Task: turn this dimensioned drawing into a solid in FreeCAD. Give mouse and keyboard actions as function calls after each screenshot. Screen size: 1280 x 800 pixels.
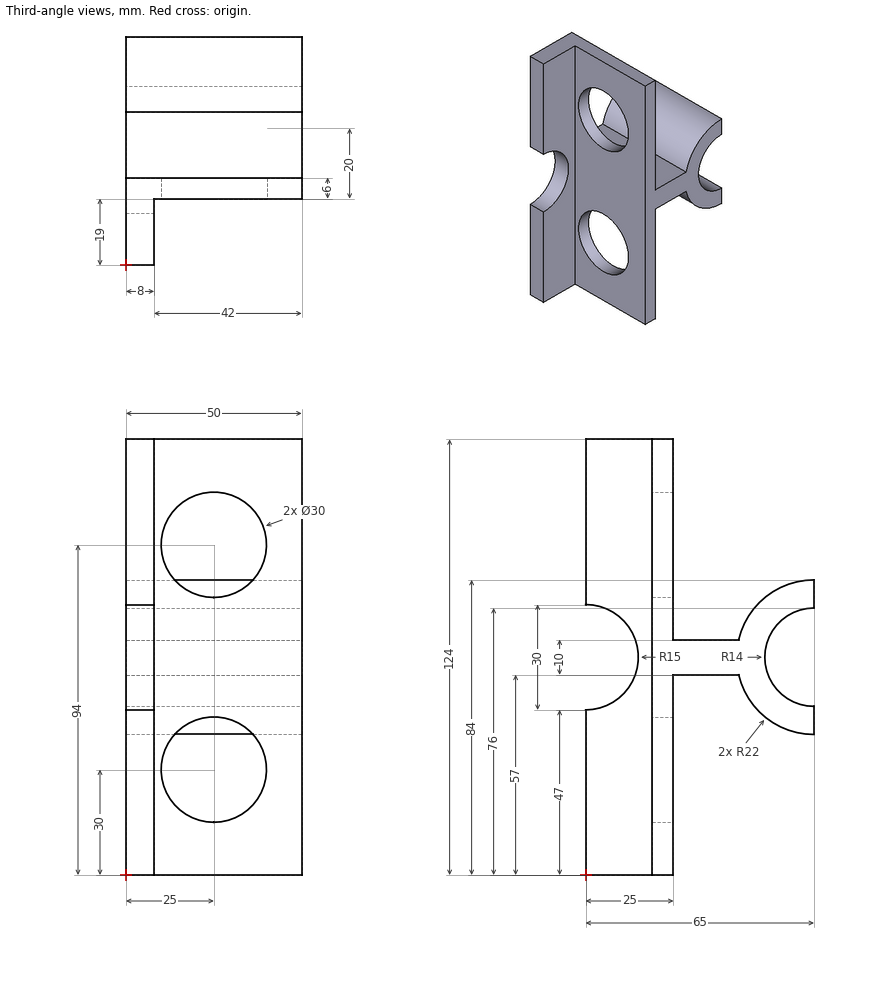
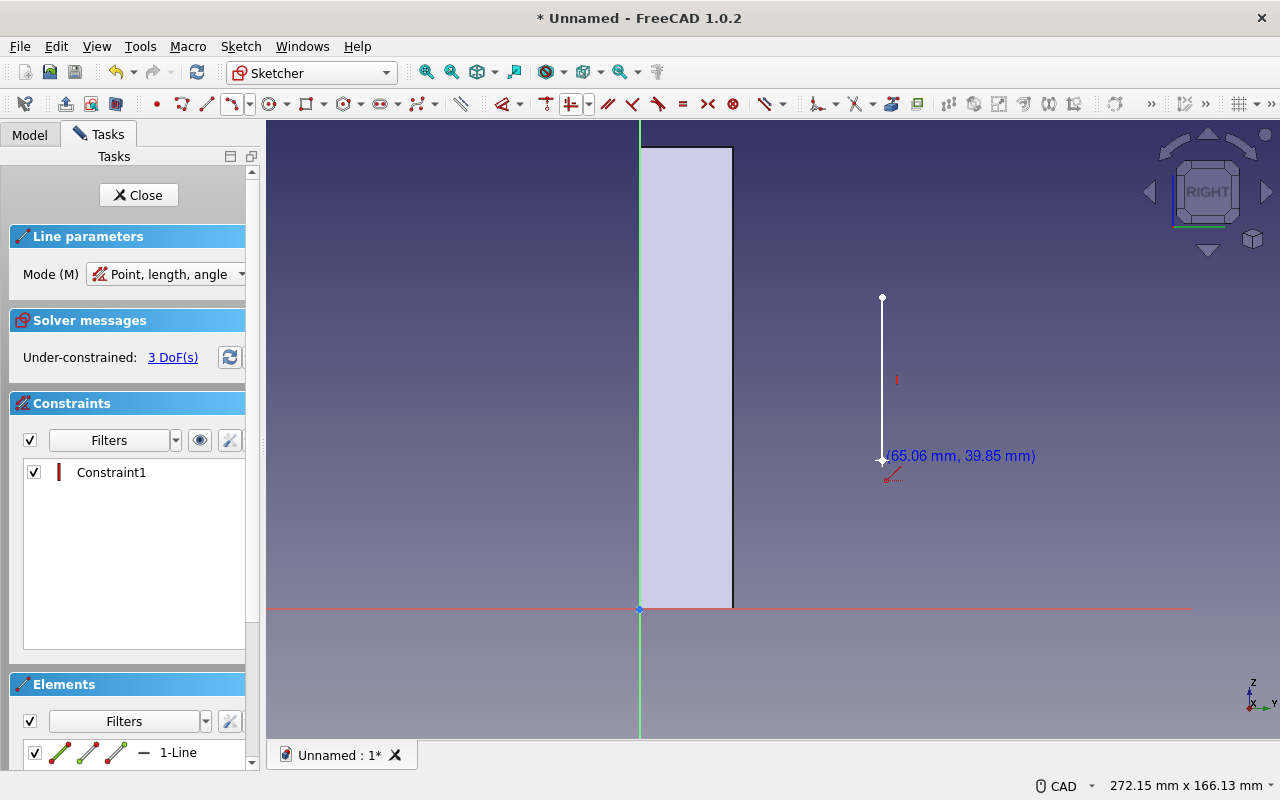
key(g)
key(m)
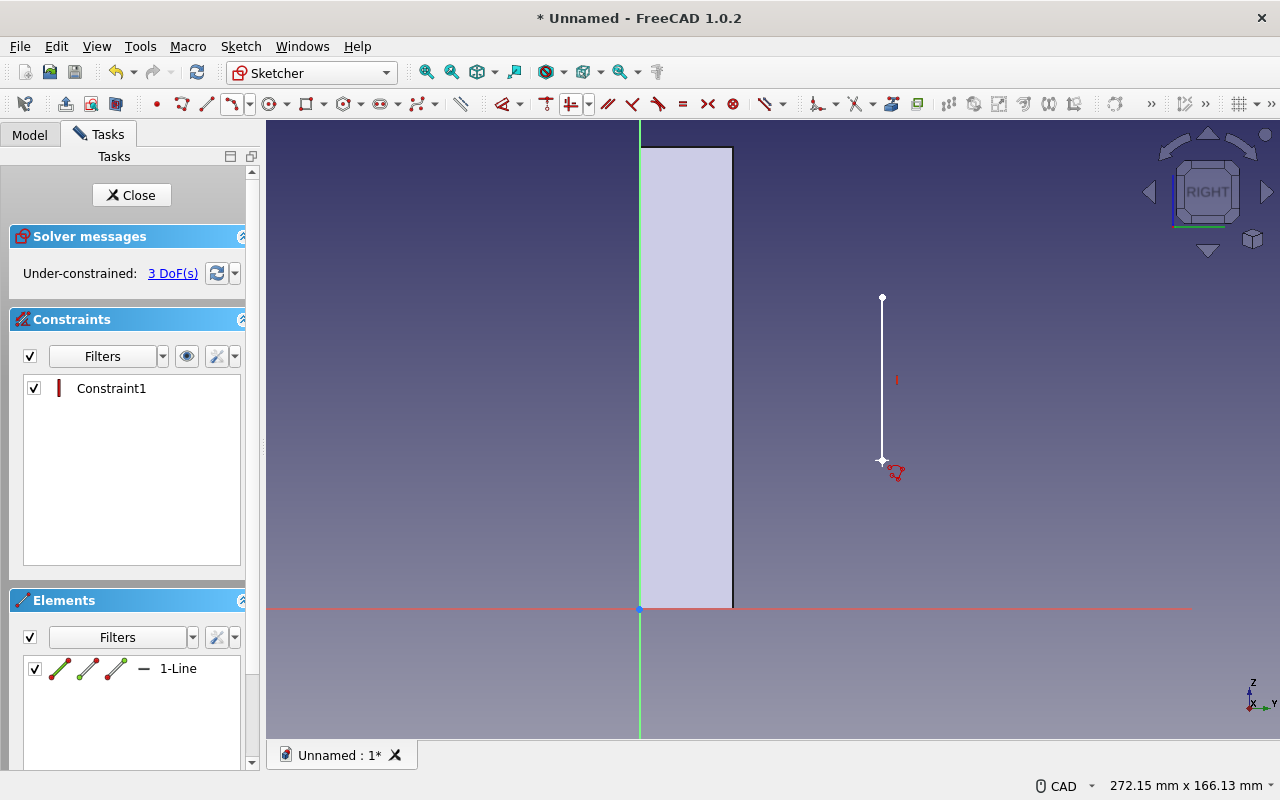
click(802, 397)
click(733, 397)
click(733, 360)
click(802, 360)
right_click(802, 360)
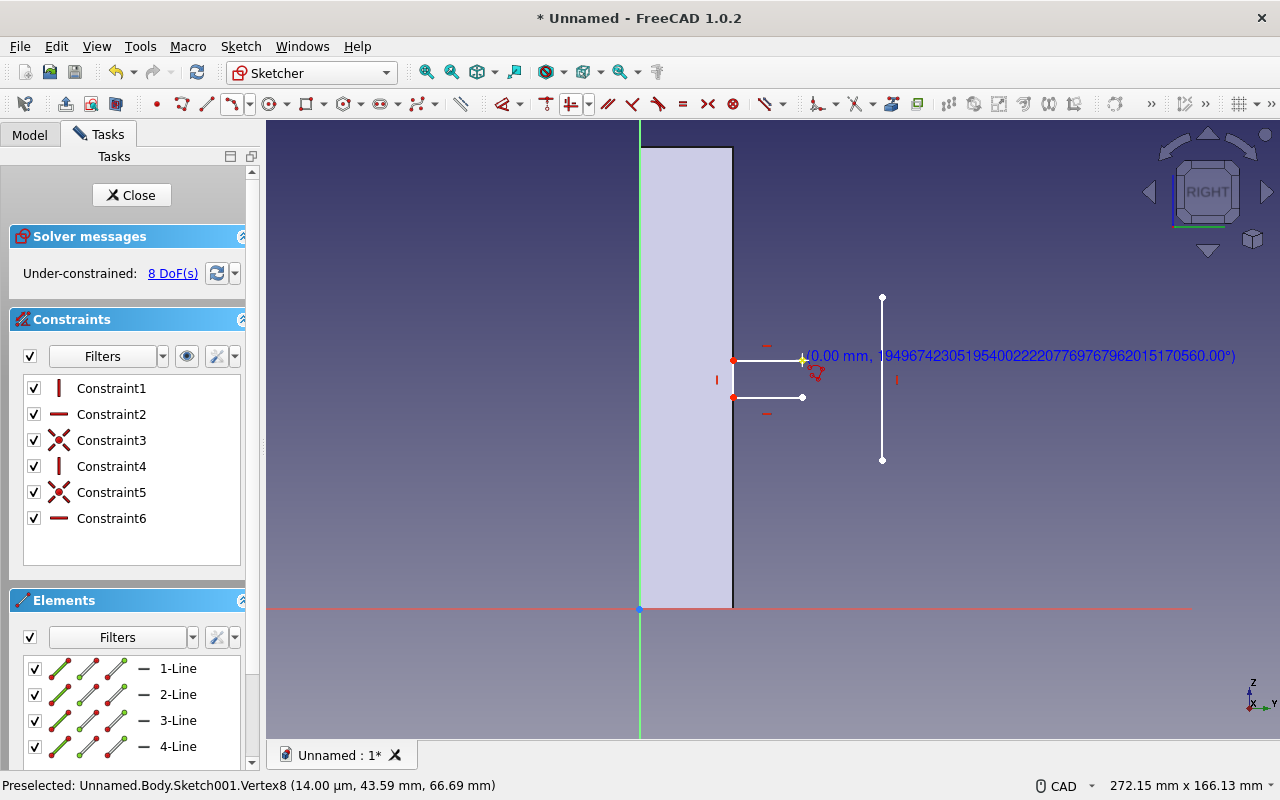
key(g)
key(3)
key(a)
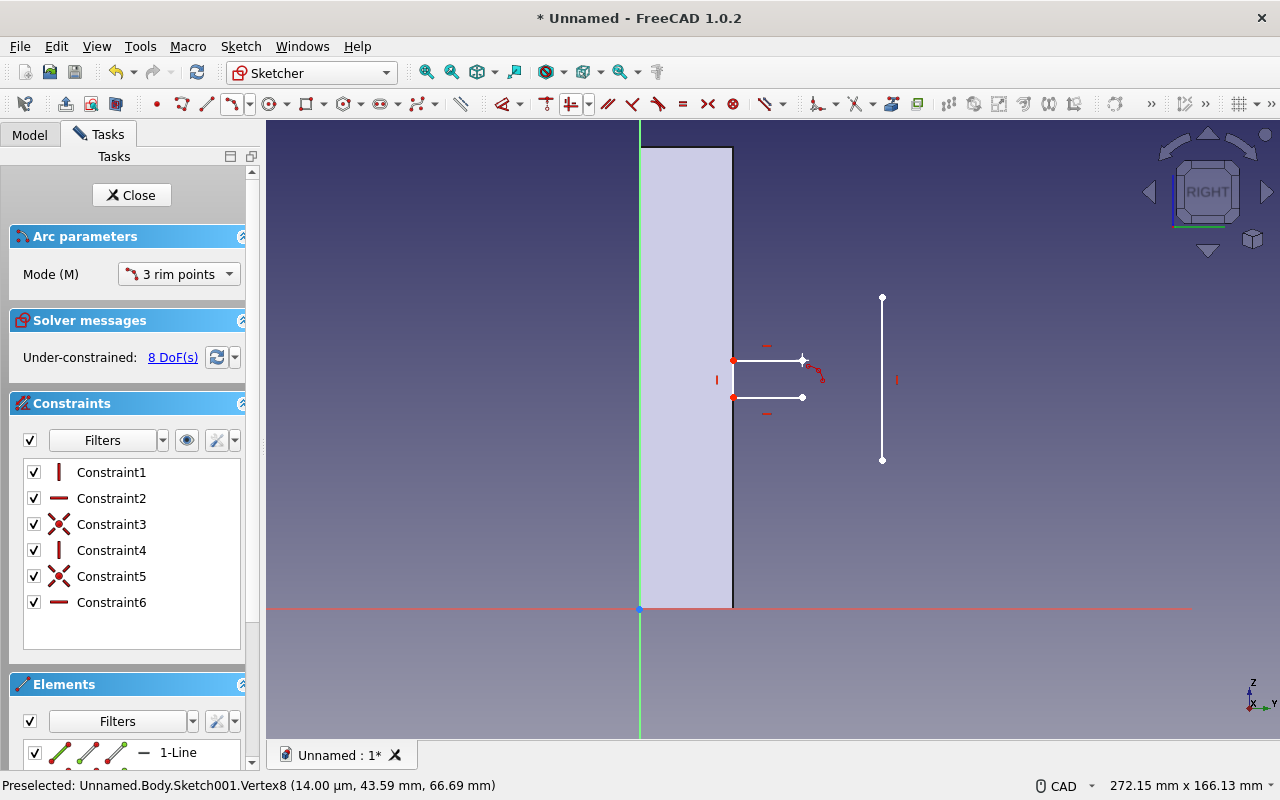
click(882, 461)
click(802, 398)
click(831, 443)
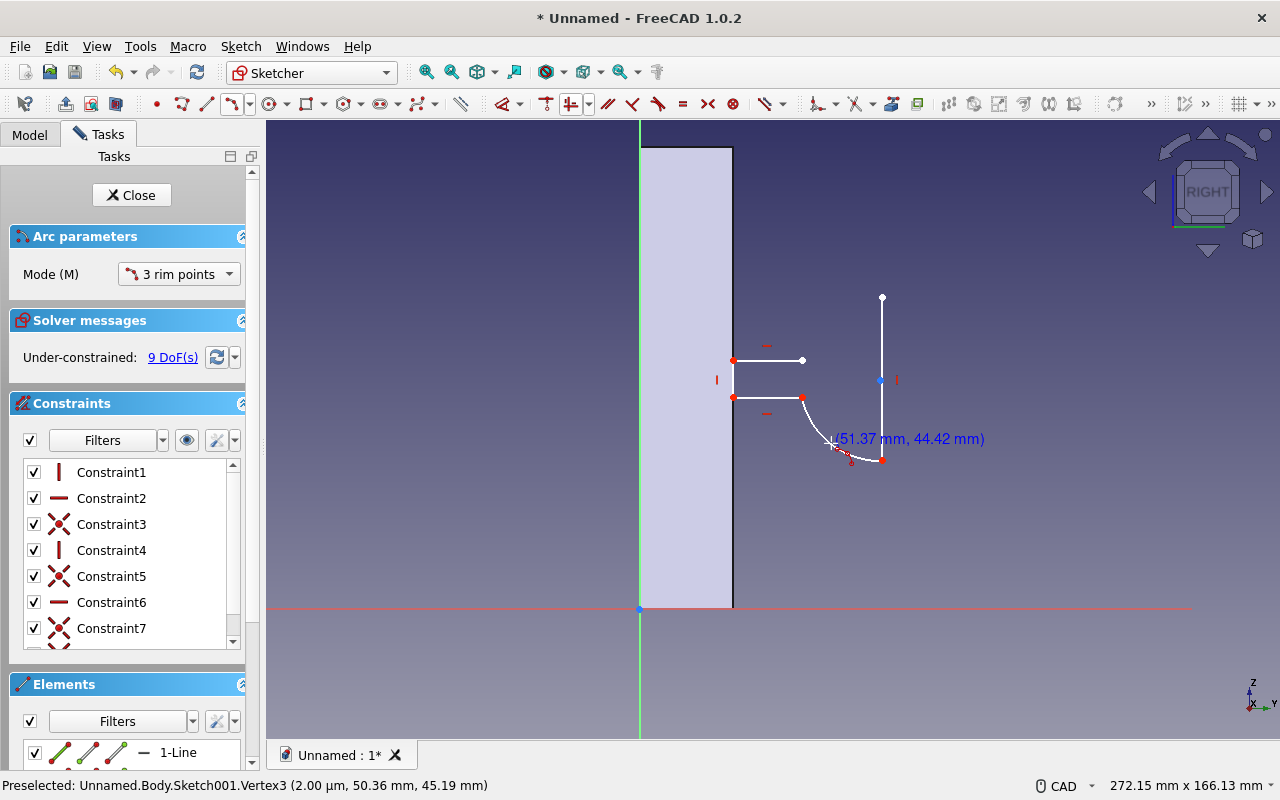
click(802, 361)
click(882, 298)
click(831, 314)
key(Escape)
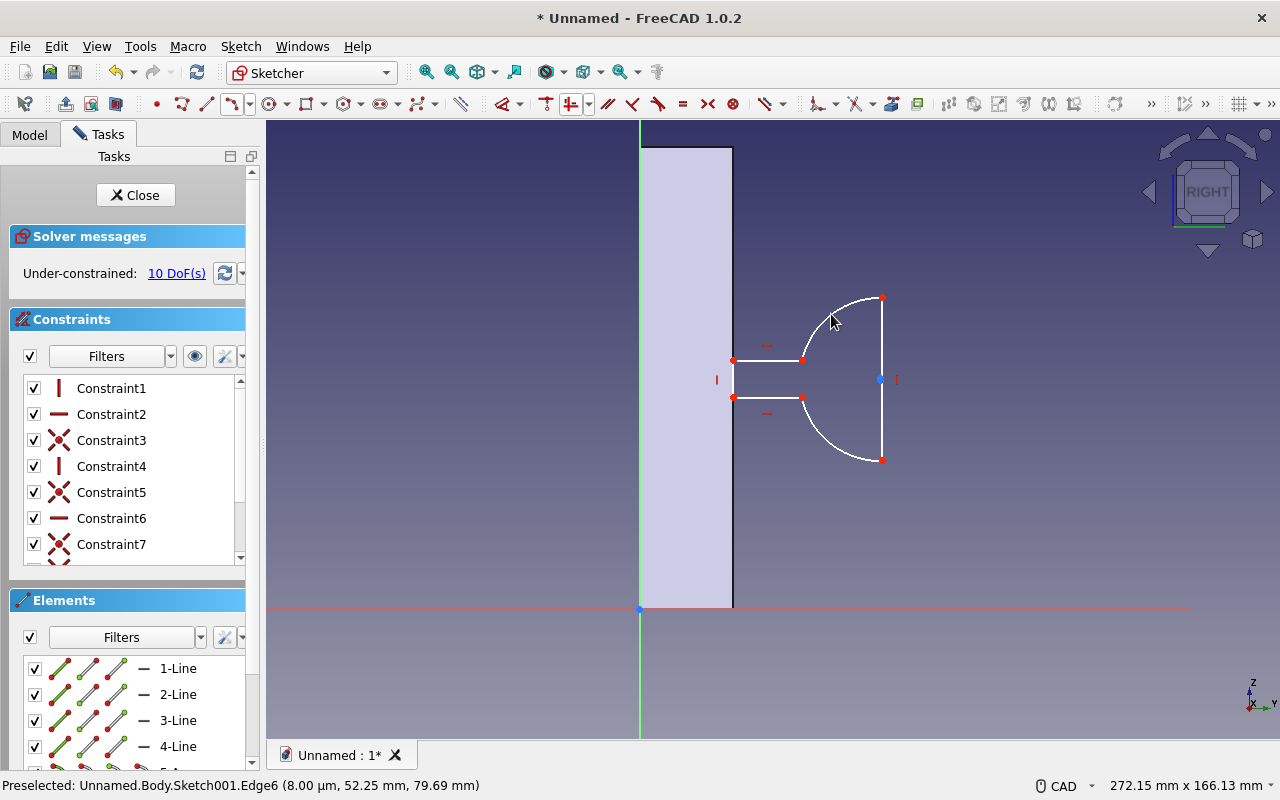
click(815, 428)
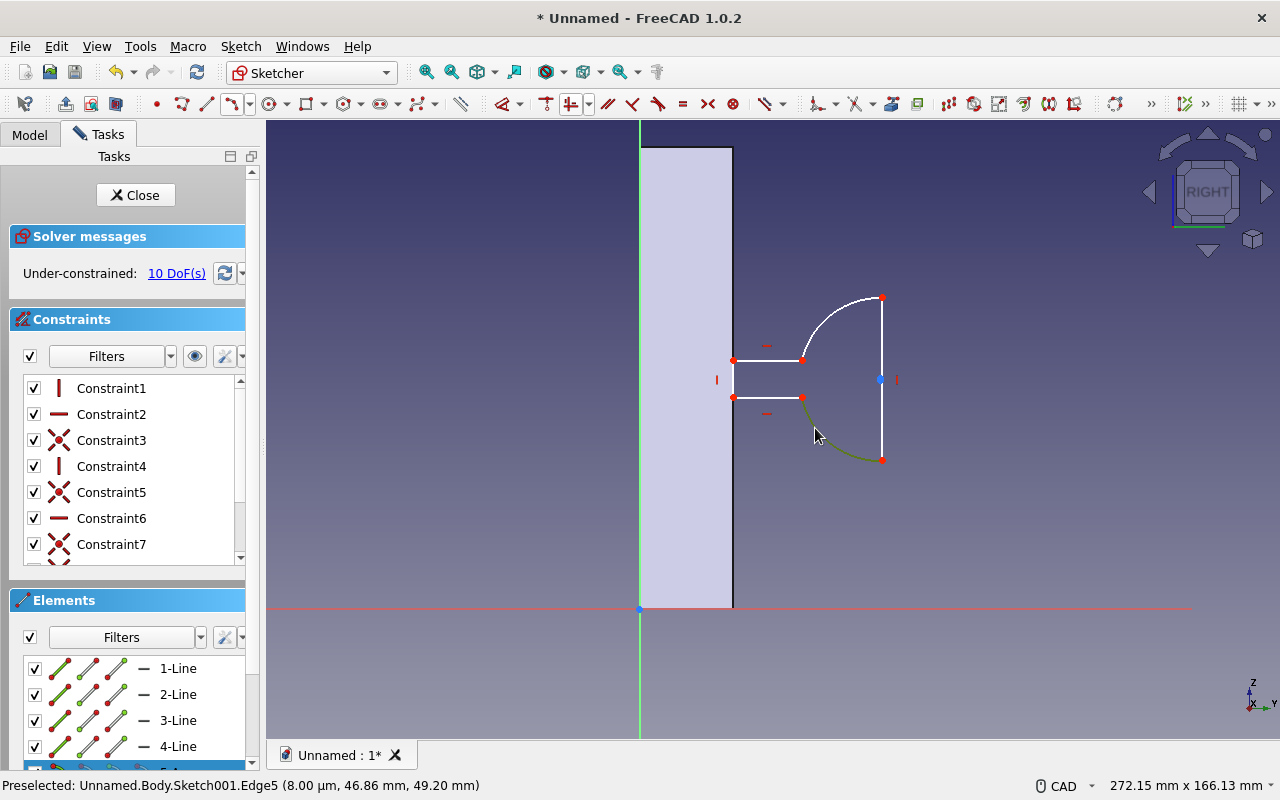
click(850, 304)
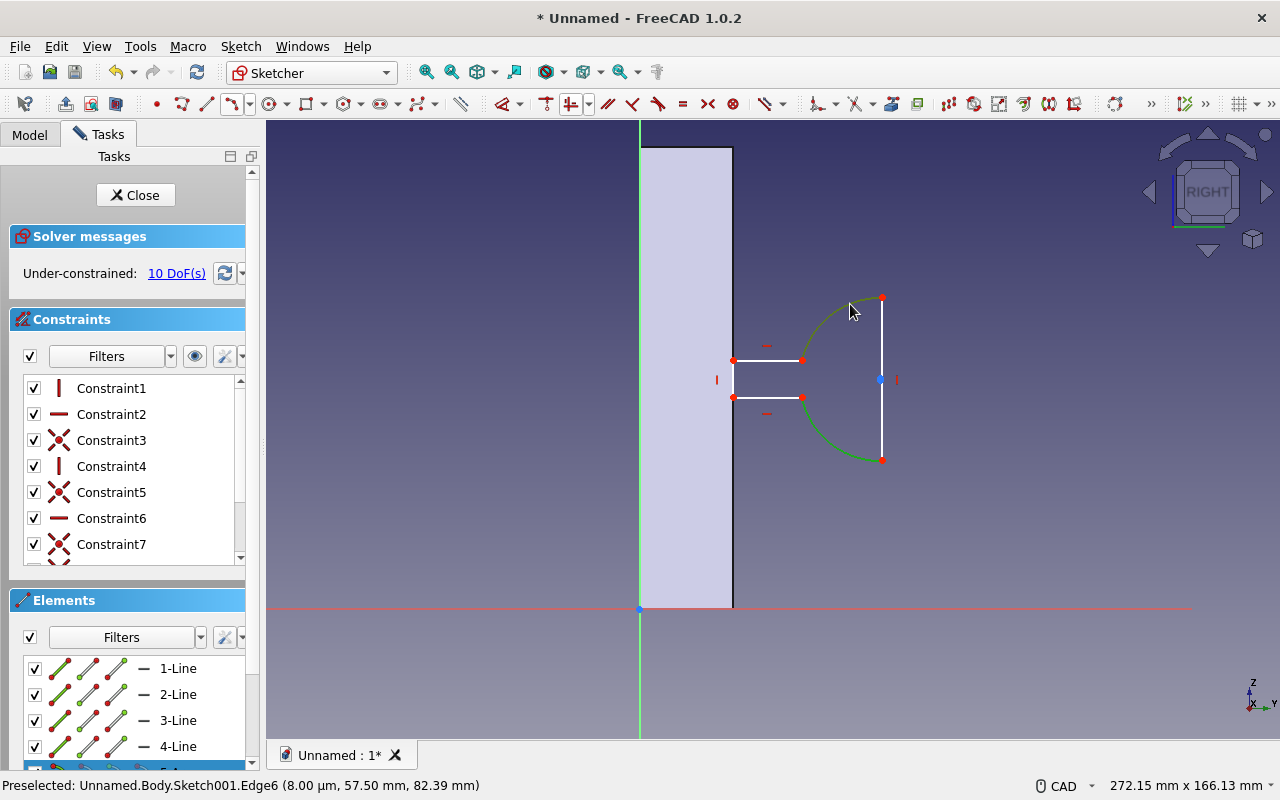
key(c)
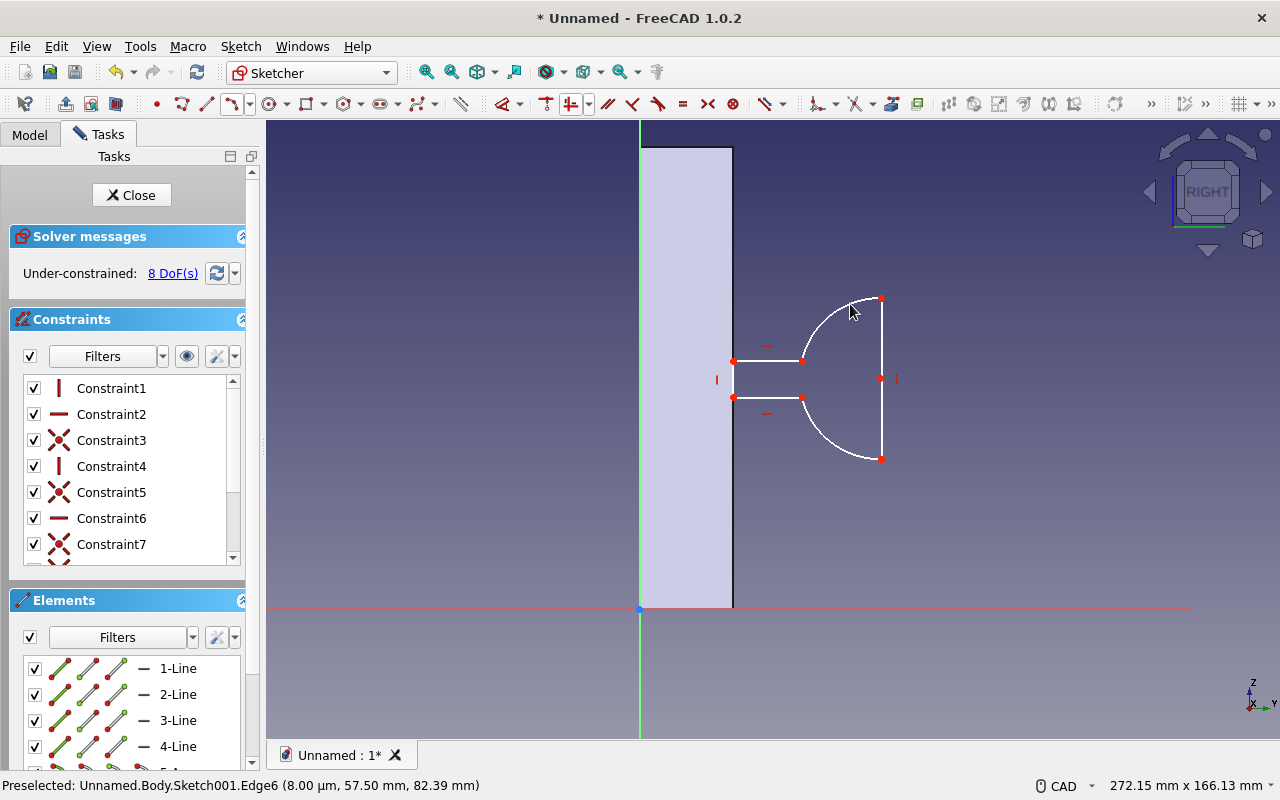
click(816, 427)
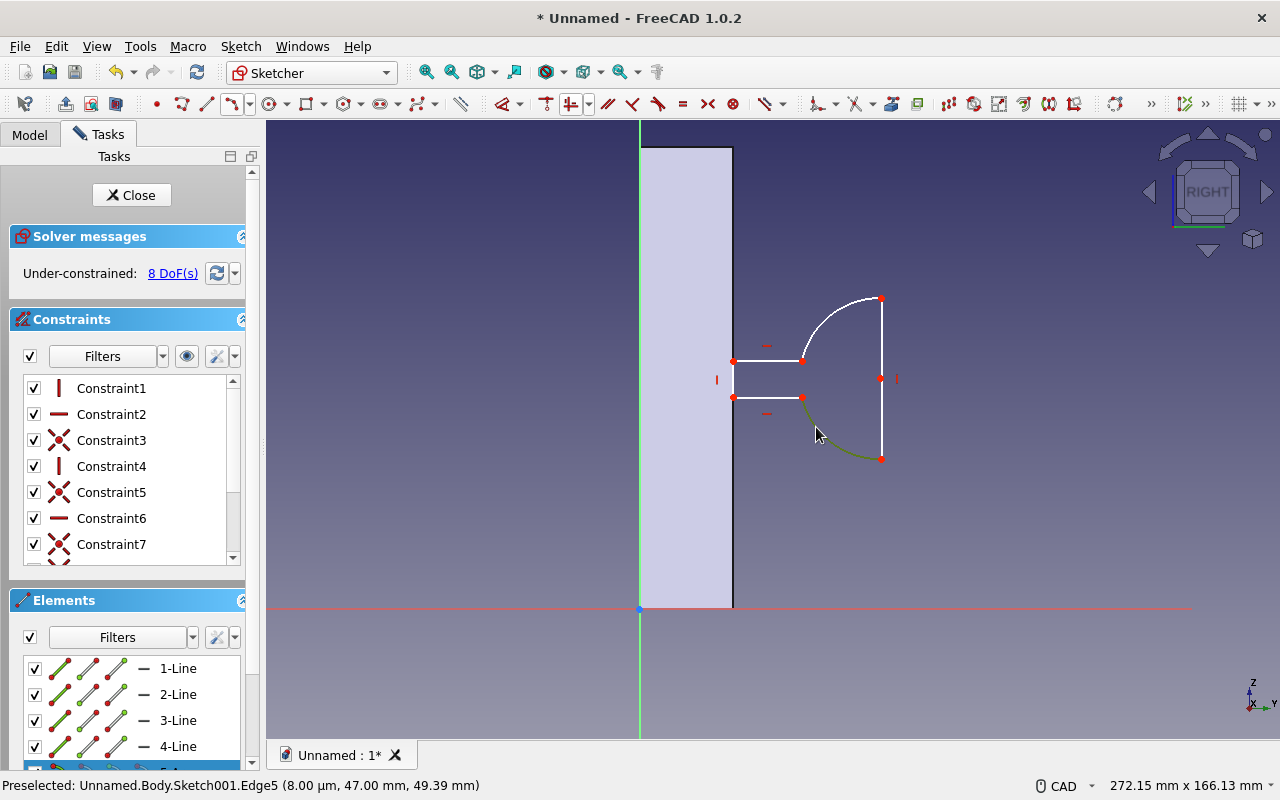
click(850, 304)